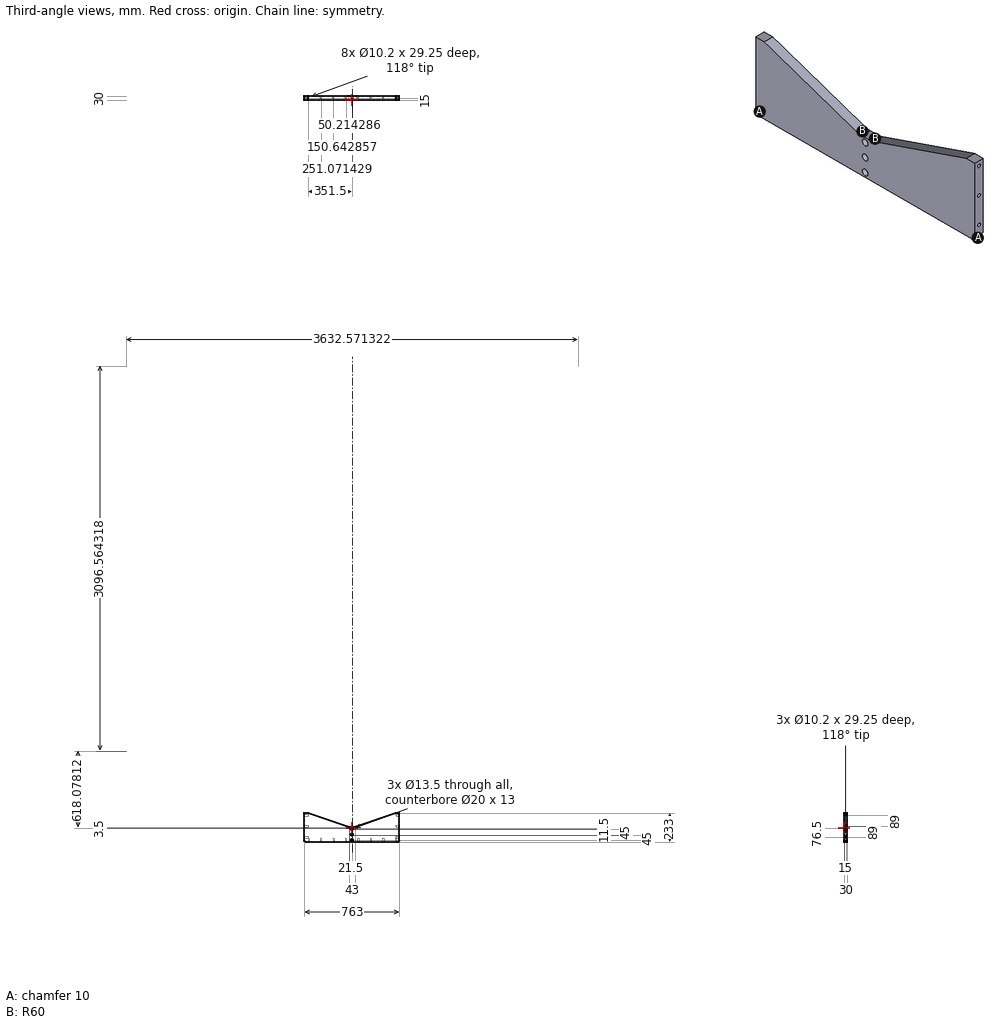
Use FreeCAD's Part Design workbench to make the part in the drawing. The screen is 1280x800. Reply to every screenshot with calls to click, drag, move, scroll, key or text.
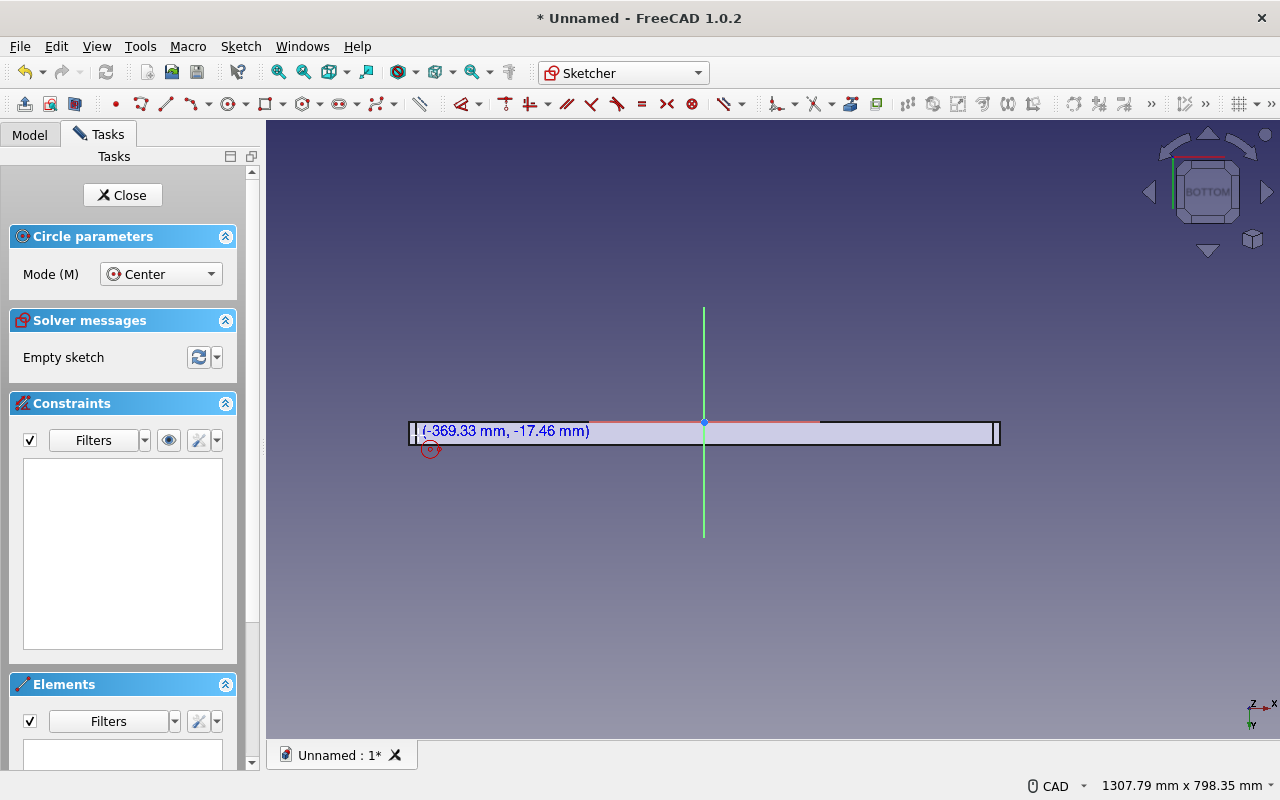
scroll(432, 434, up, 2)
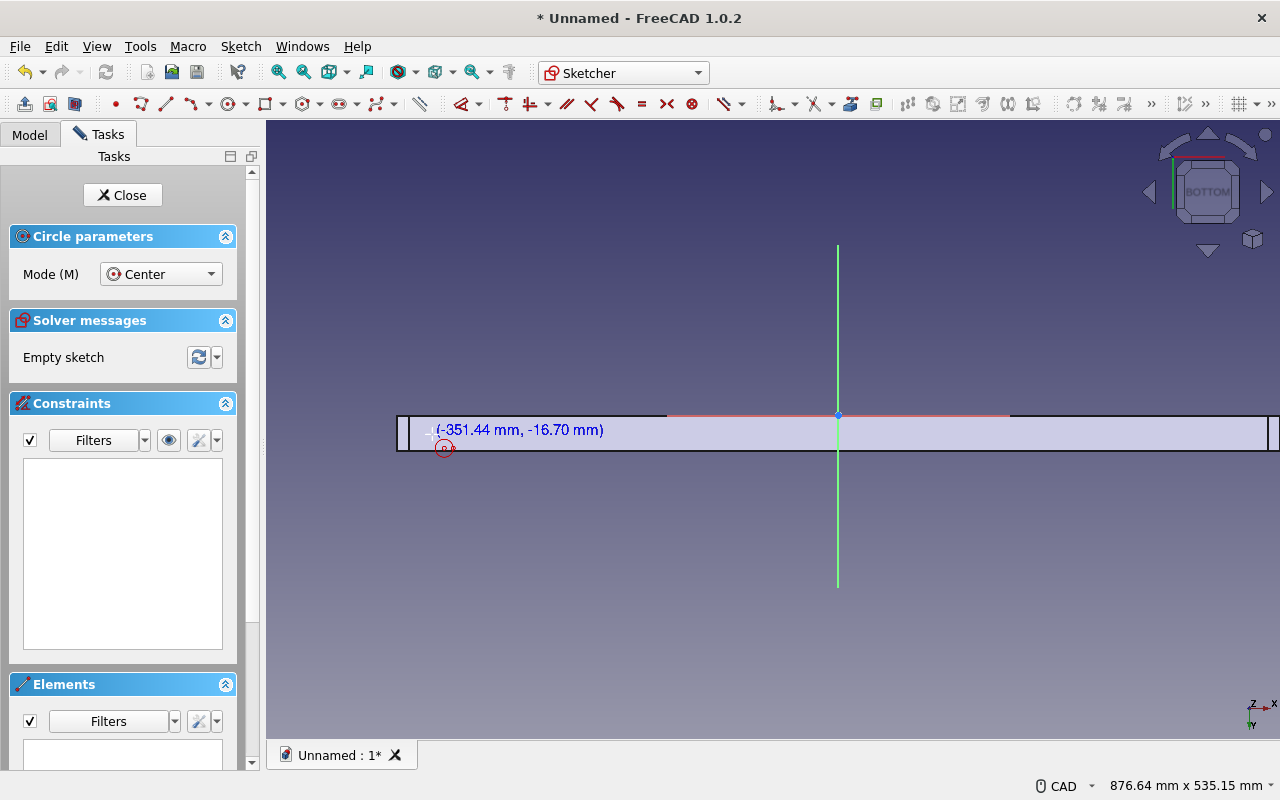
click(432, 433)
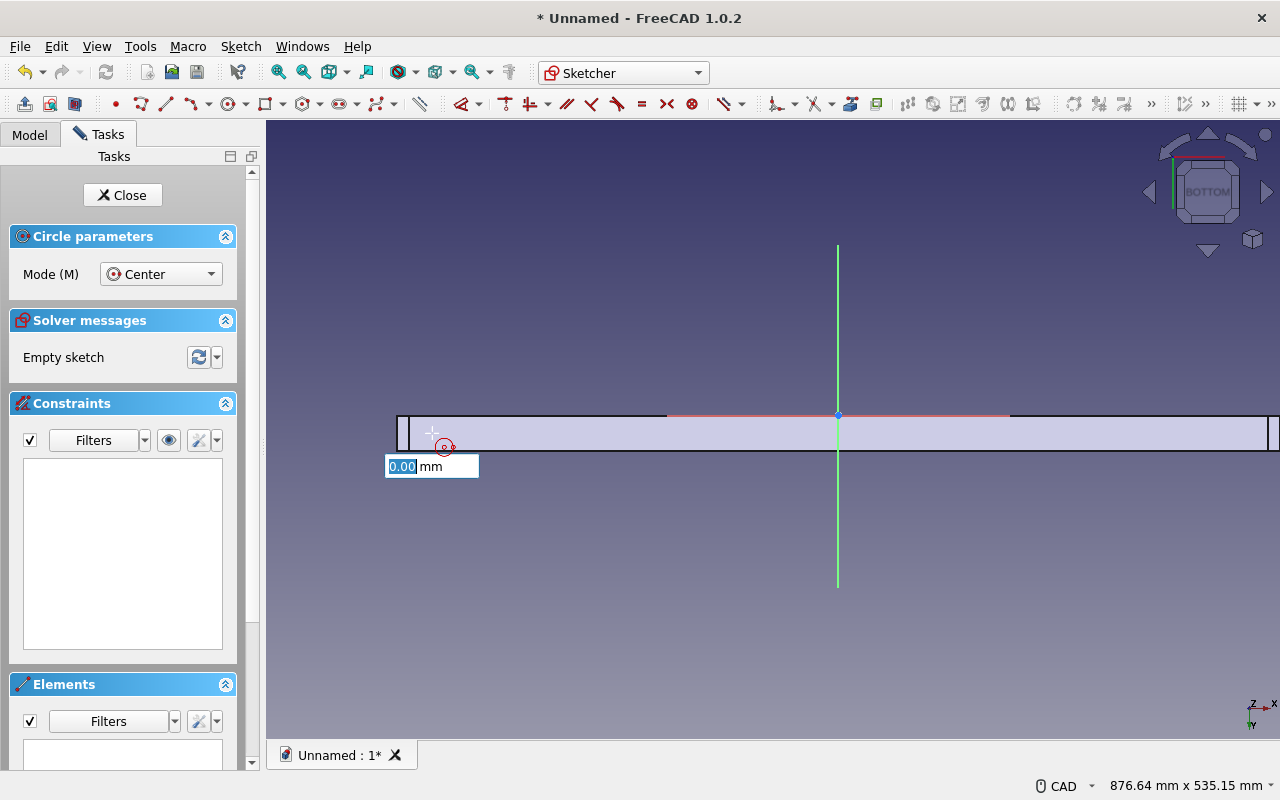
scroll(436, 437, up, 5)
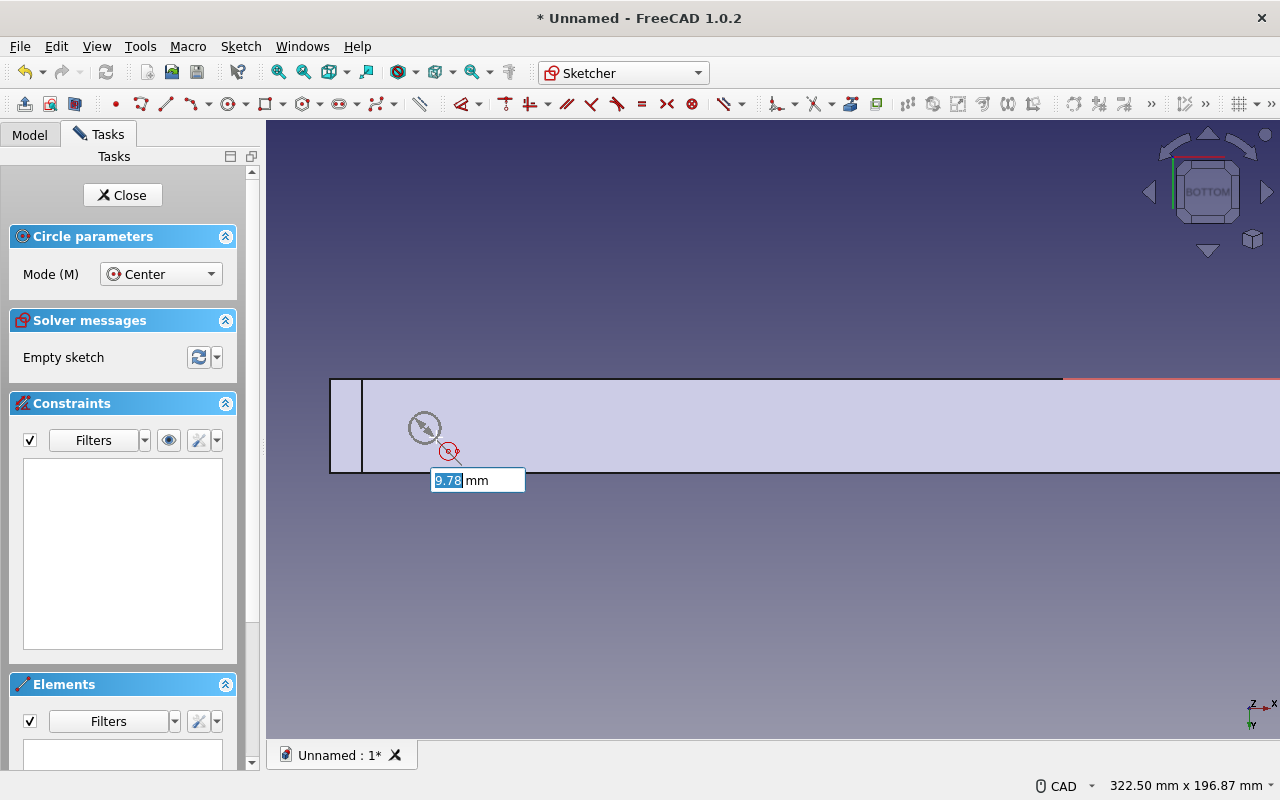
click(436, 437)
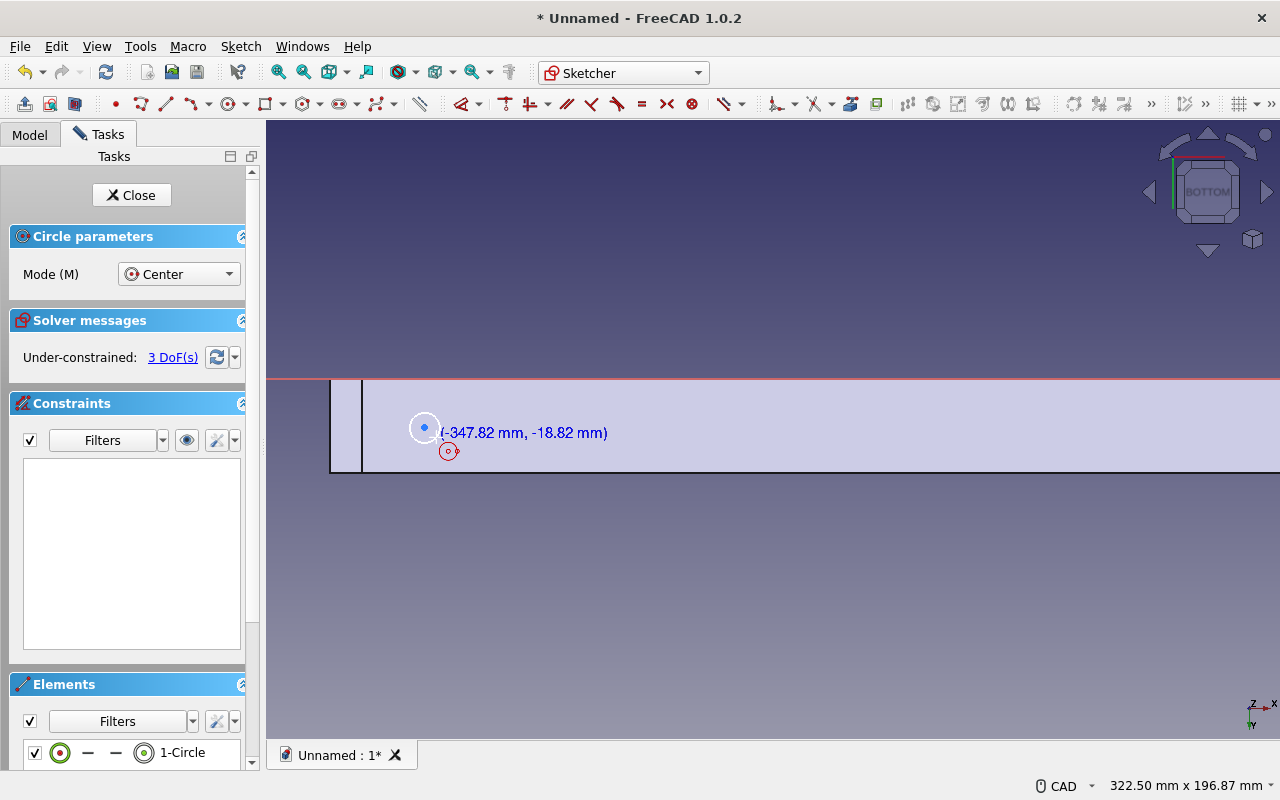
scroll(740, 426, up, 2)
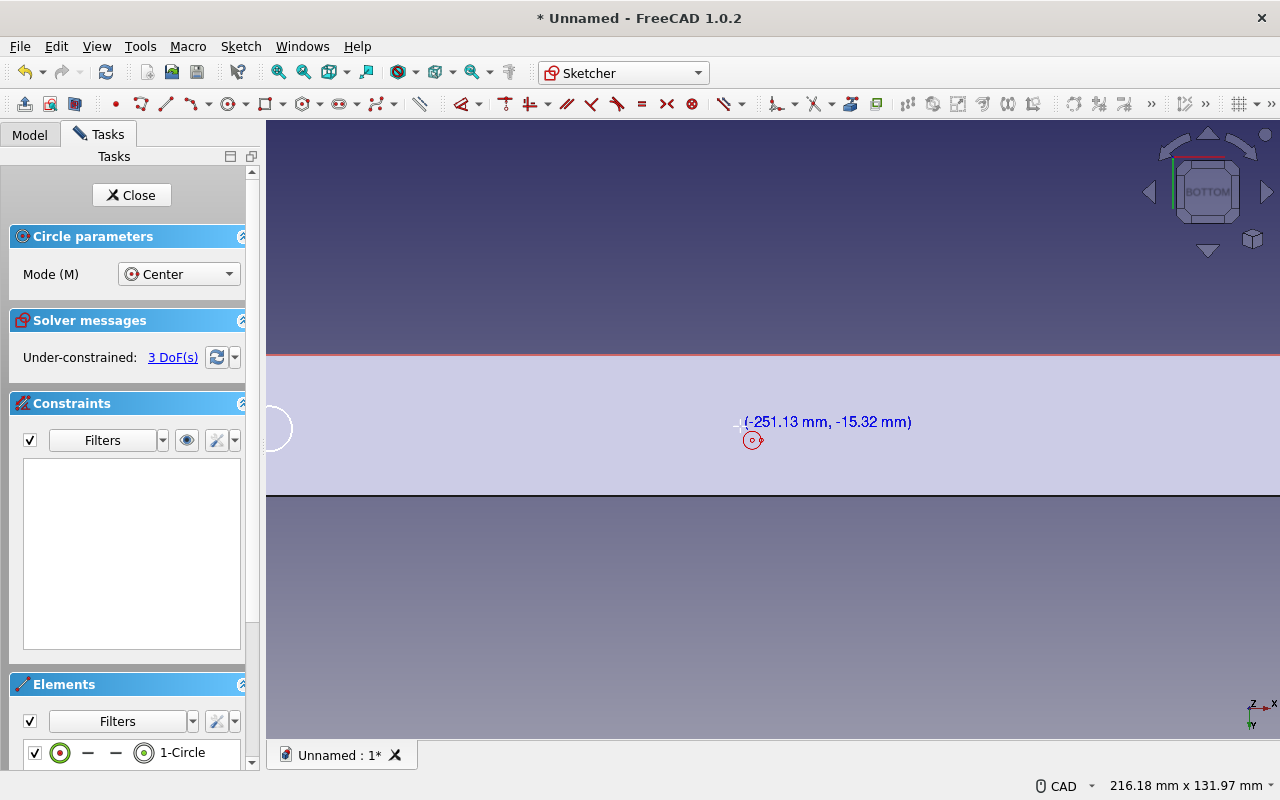
scroll(464, 435, down, 9)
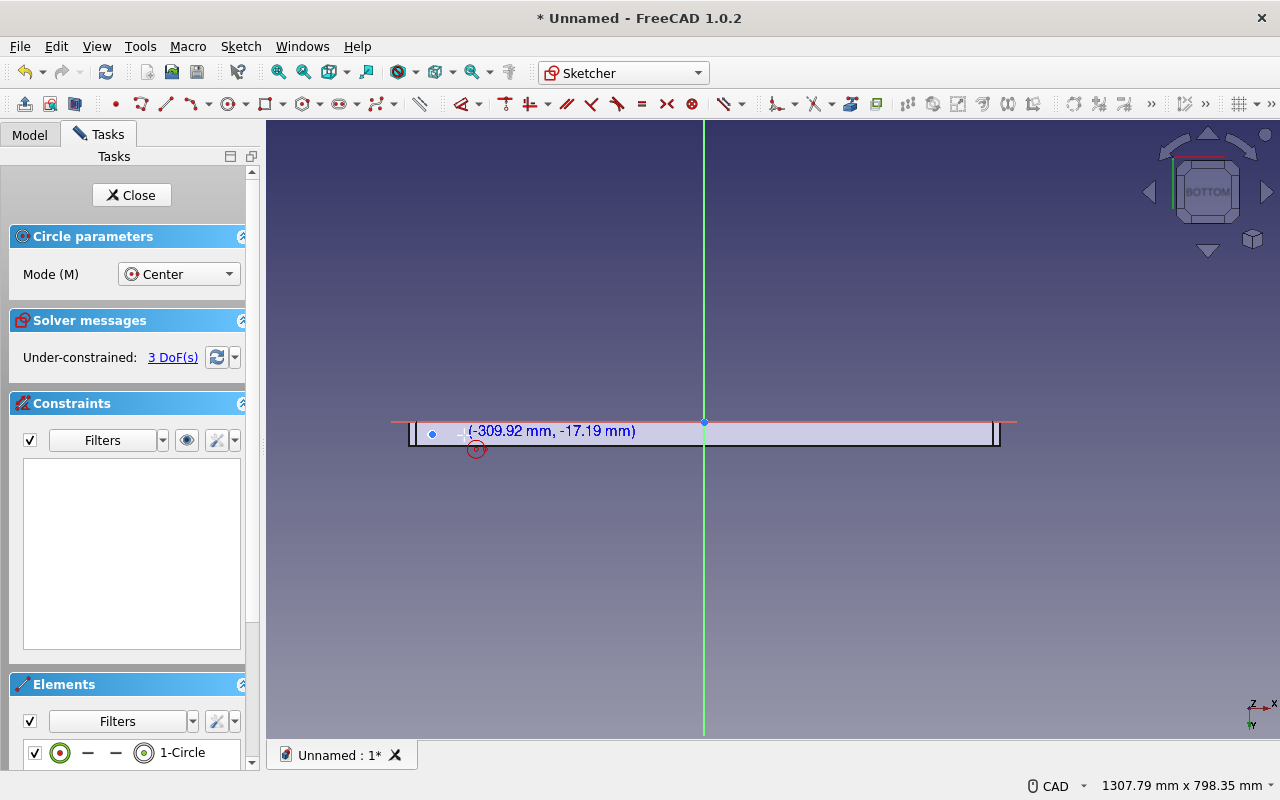
scroll(510, 434, up, 2)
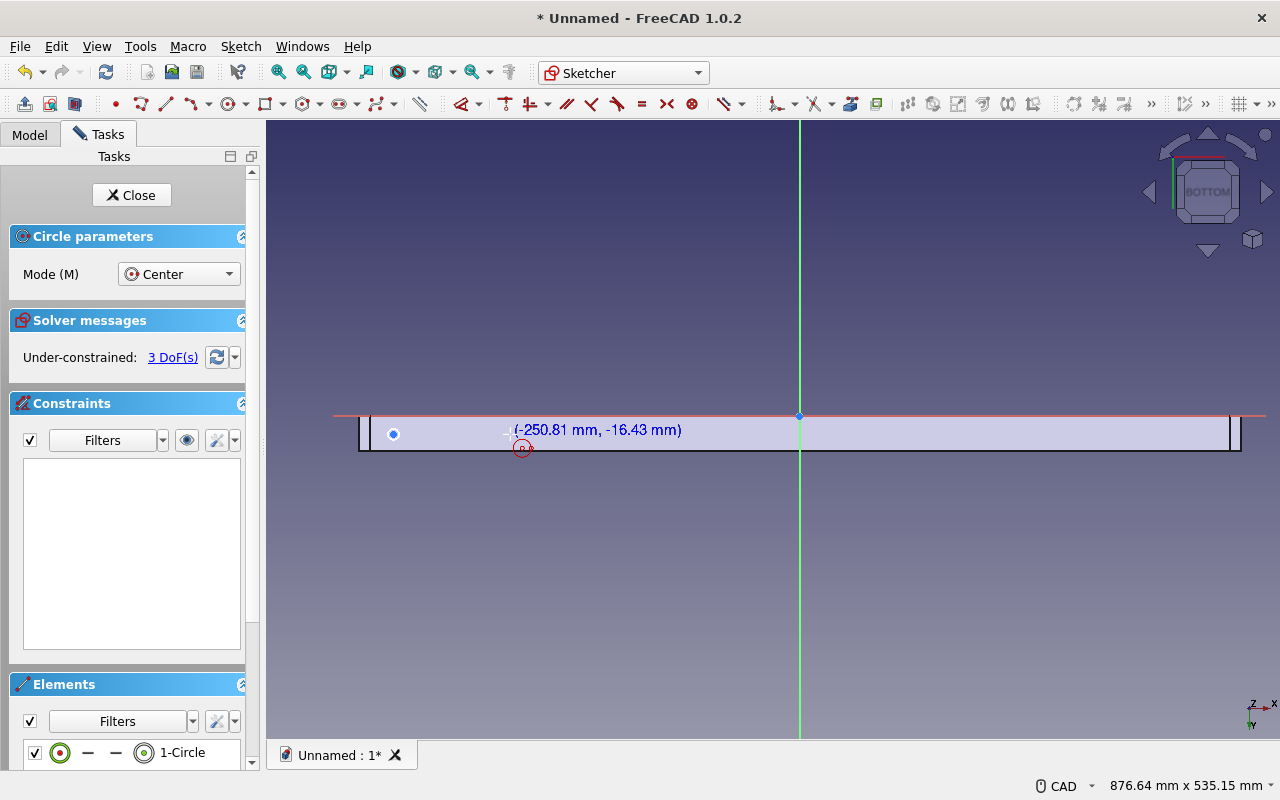
click(510, 434)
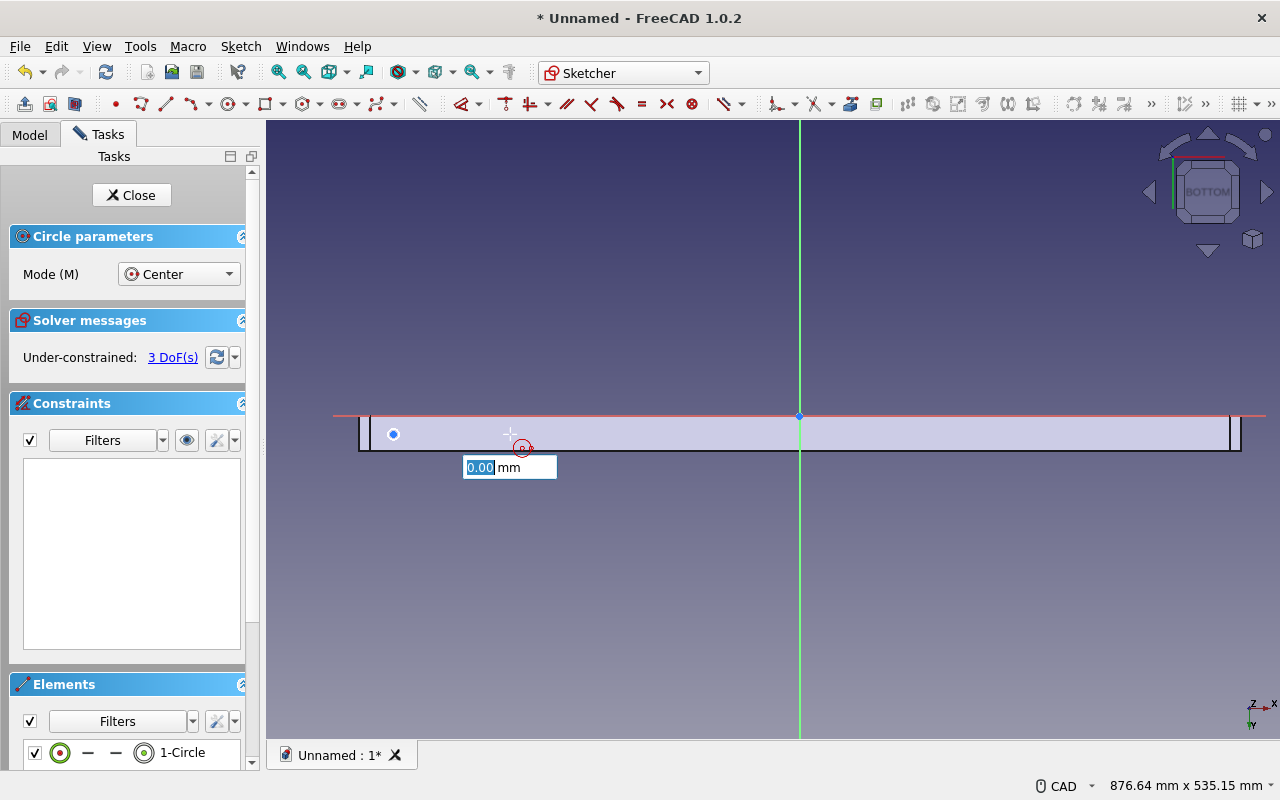
scroll(514, 438, up, 5)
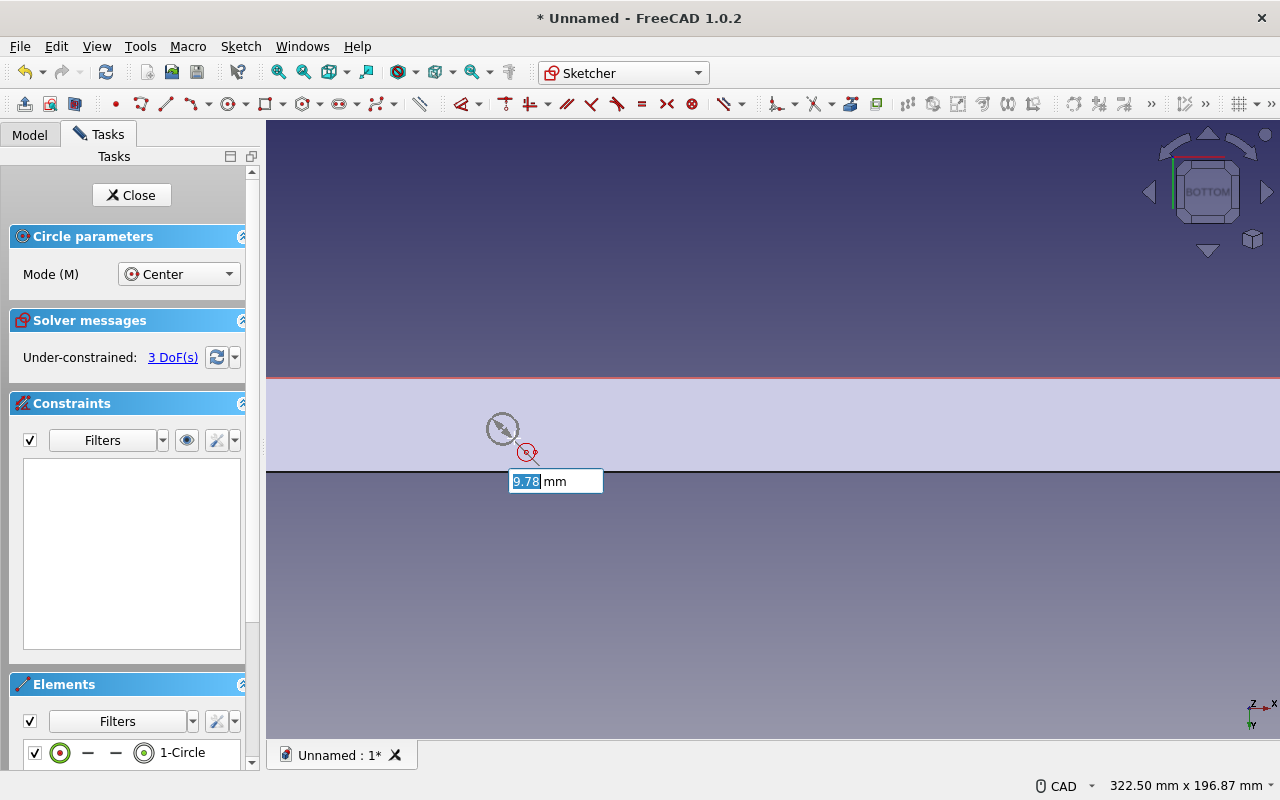
click(513, 436)